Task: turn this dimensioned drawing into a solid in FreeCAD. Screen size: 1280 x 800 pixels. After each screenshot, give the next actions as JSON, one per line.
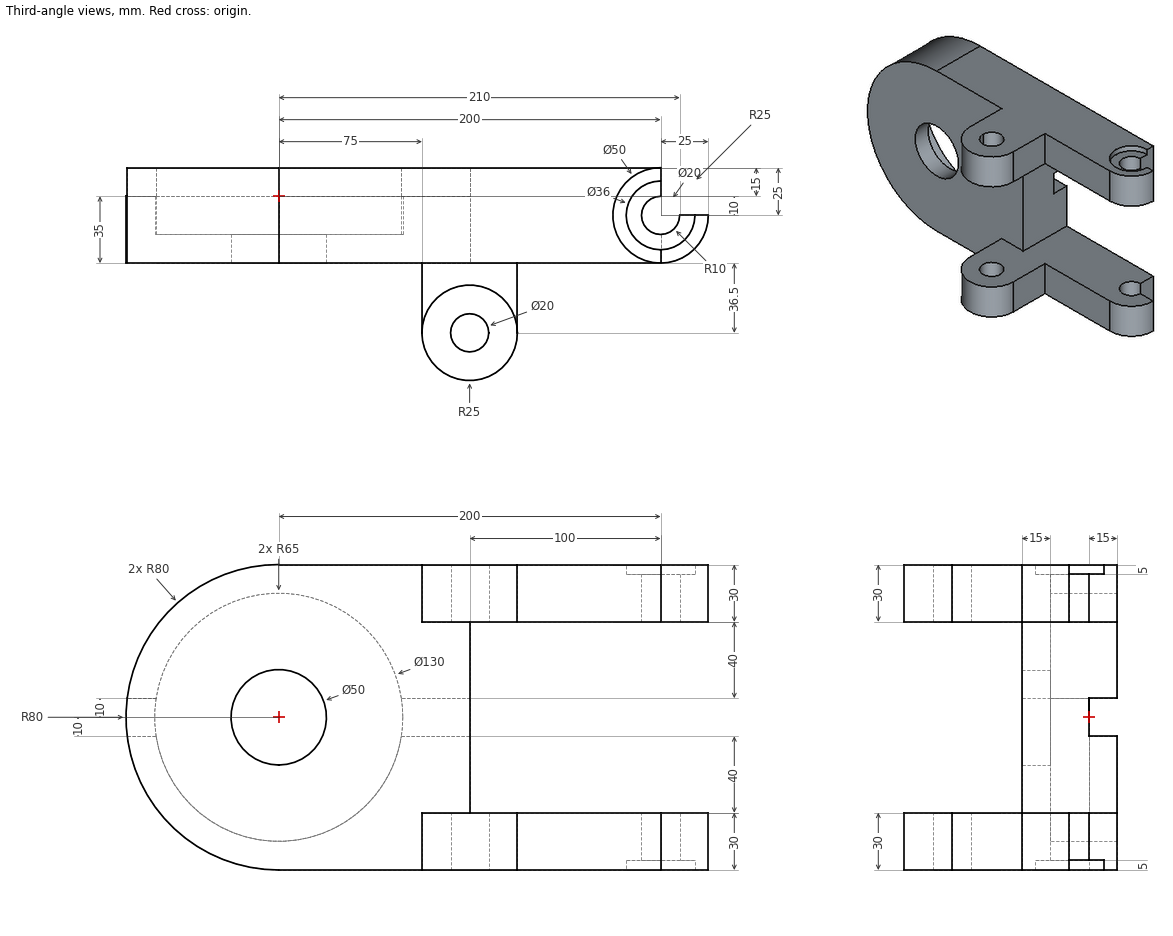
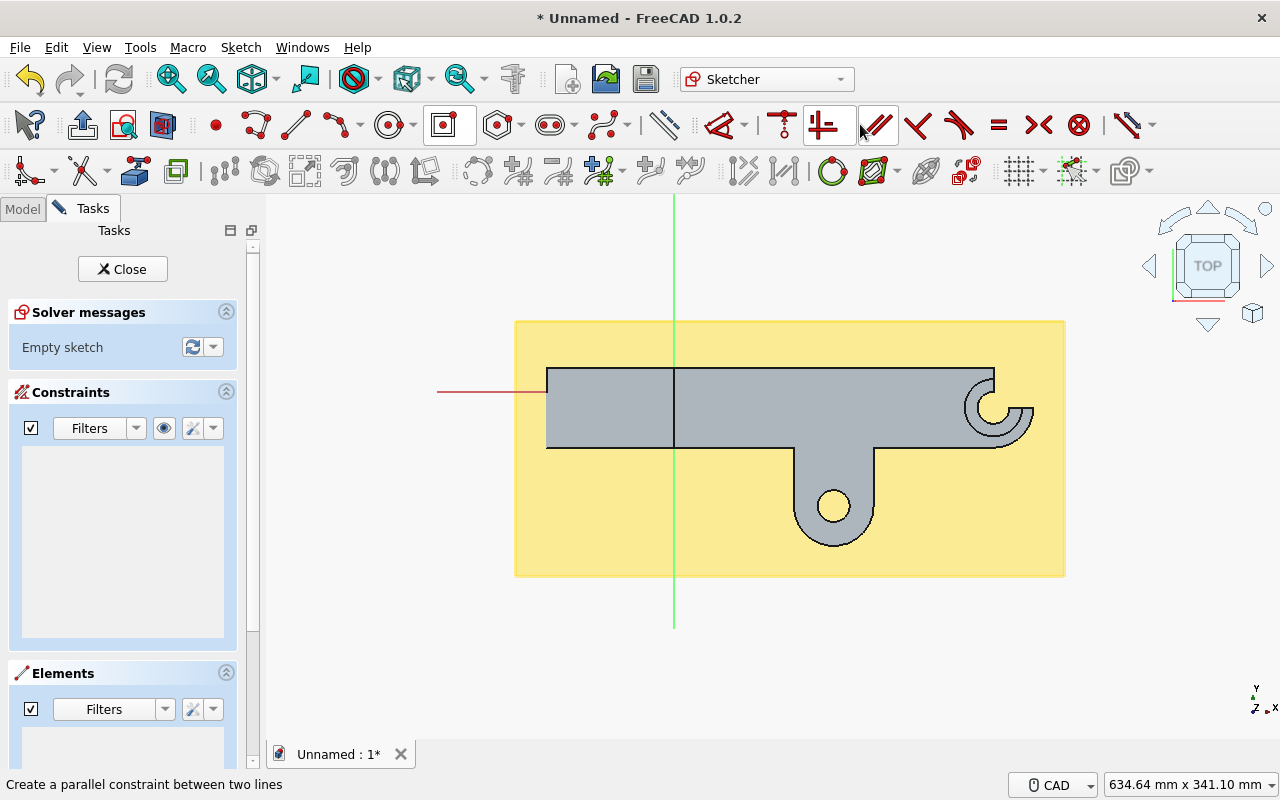
{"action": "key", "text": "q s"}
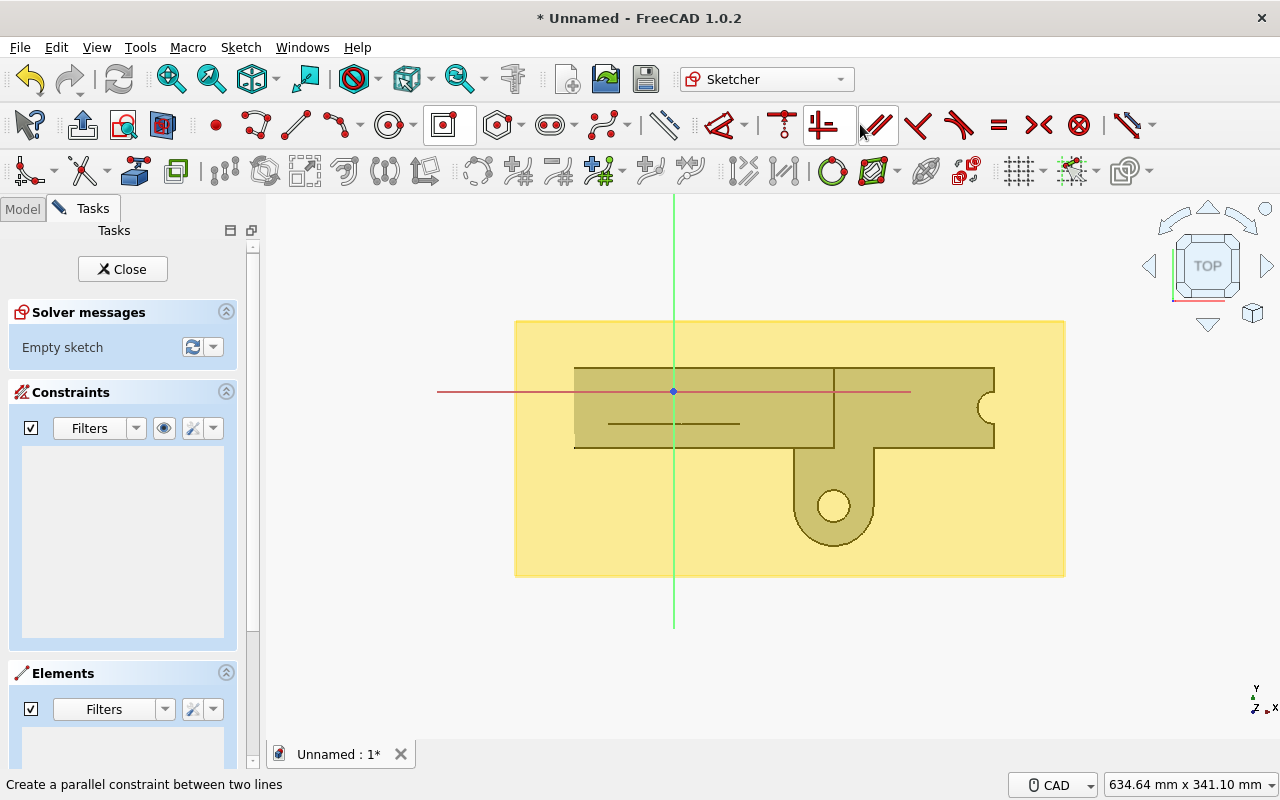
{"action": "scroll", "coordinate": [1052, 423], "scroll_direction": "up", "scroll_amount": 11}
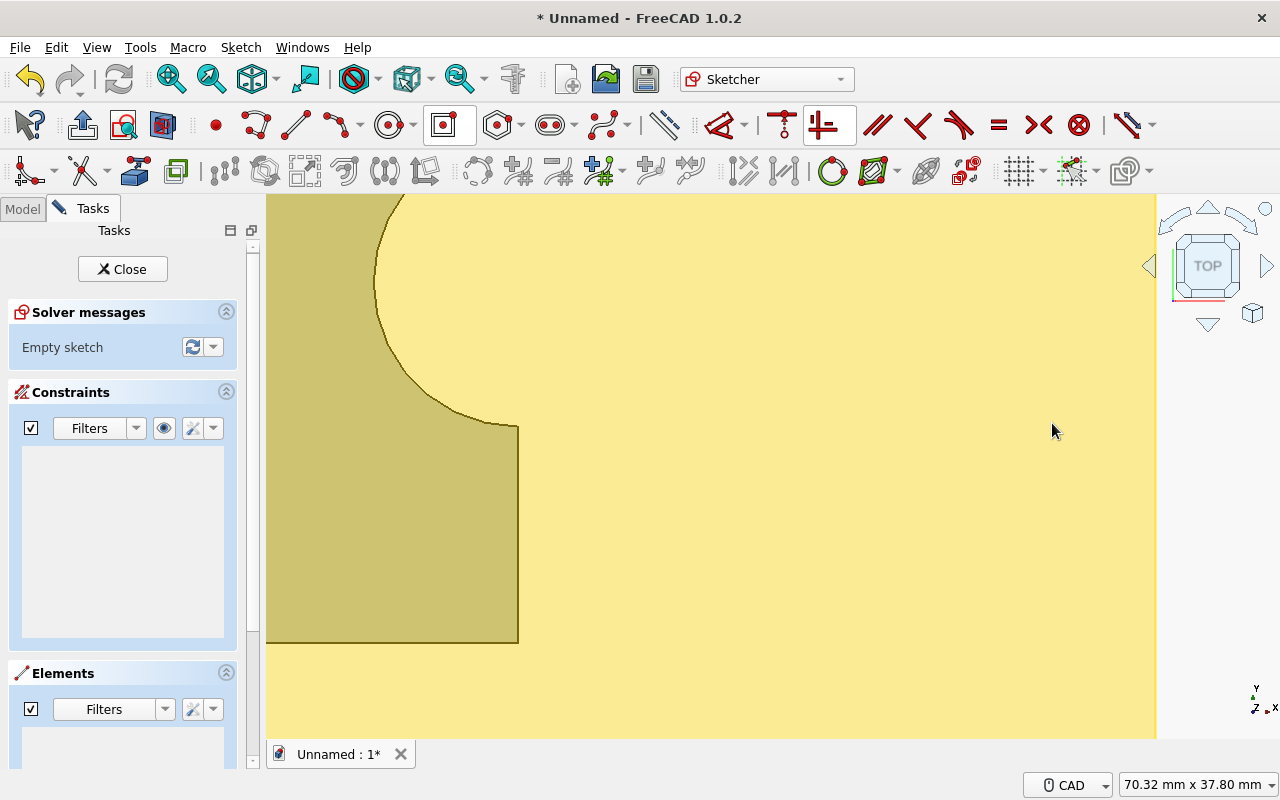
{"action": "key", "text": "g l"}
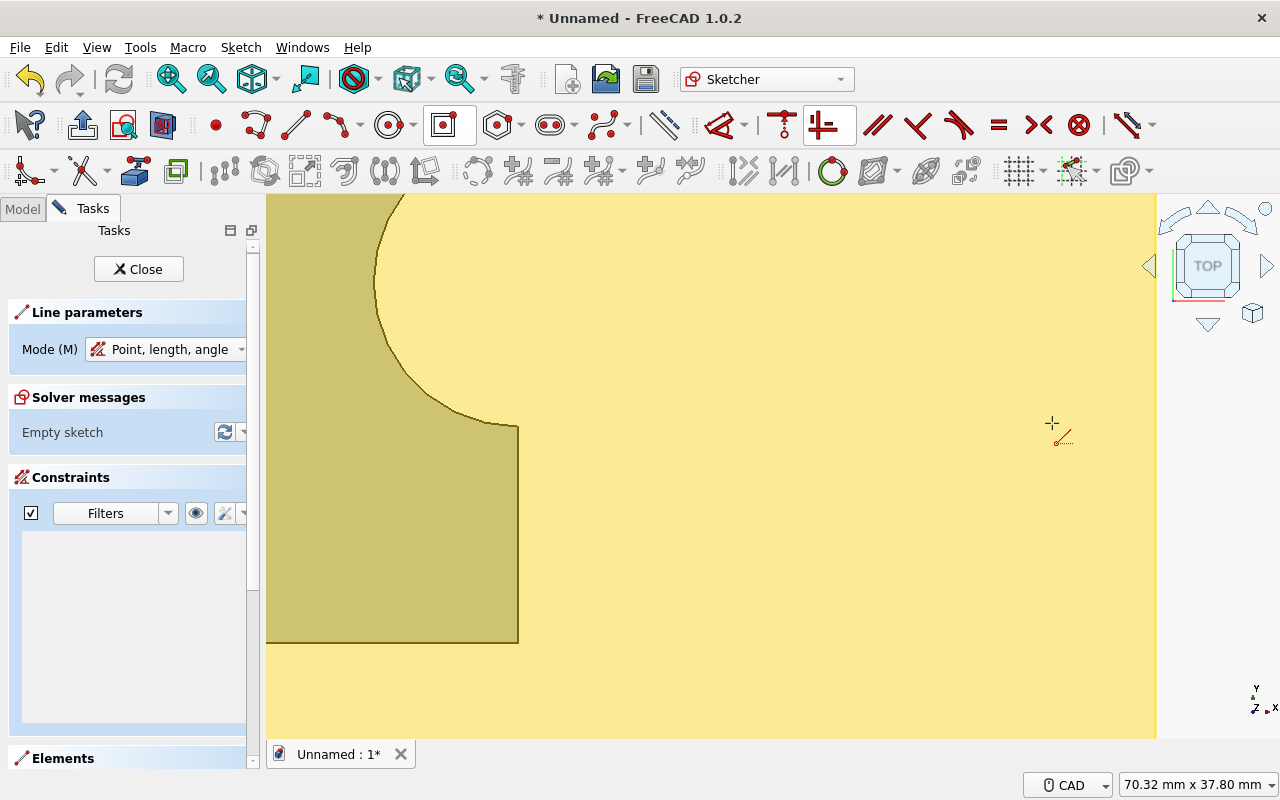
{"action": "left_click", "coordinate": [662, 282]}
{"action": "left_click", "coordinate": [878, 282]}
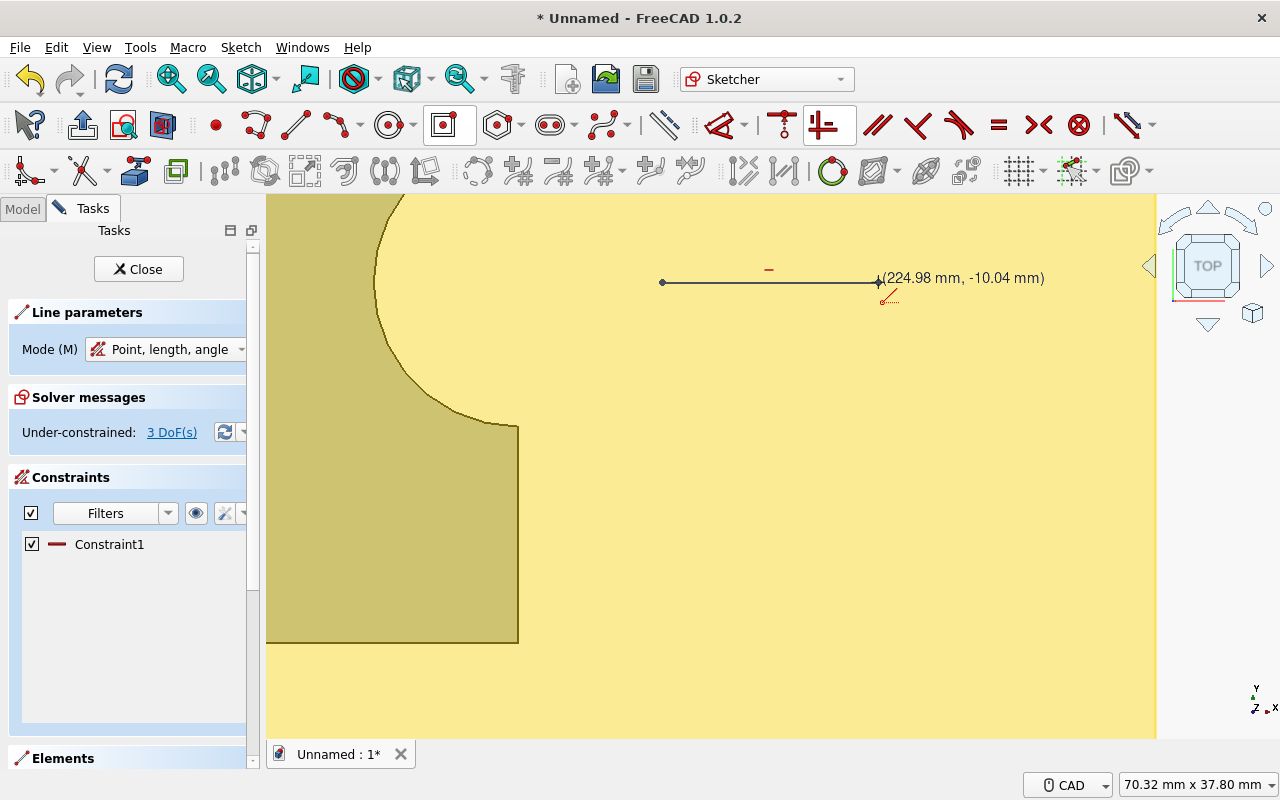
{"action": "left_click", "coordinate": [518, 643]}
{"action": "left_click", "coordinate": [518, 427]}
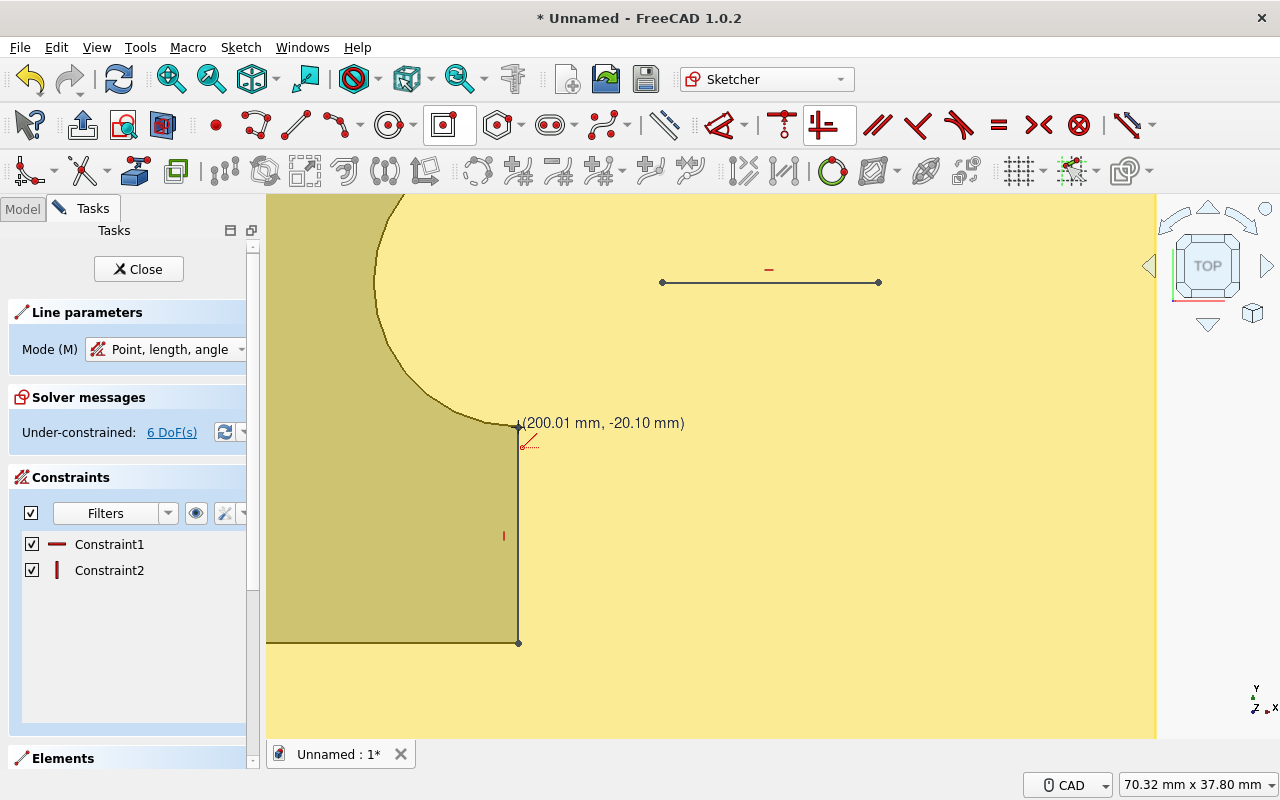
{"action": "key", "text": "g 3 a"}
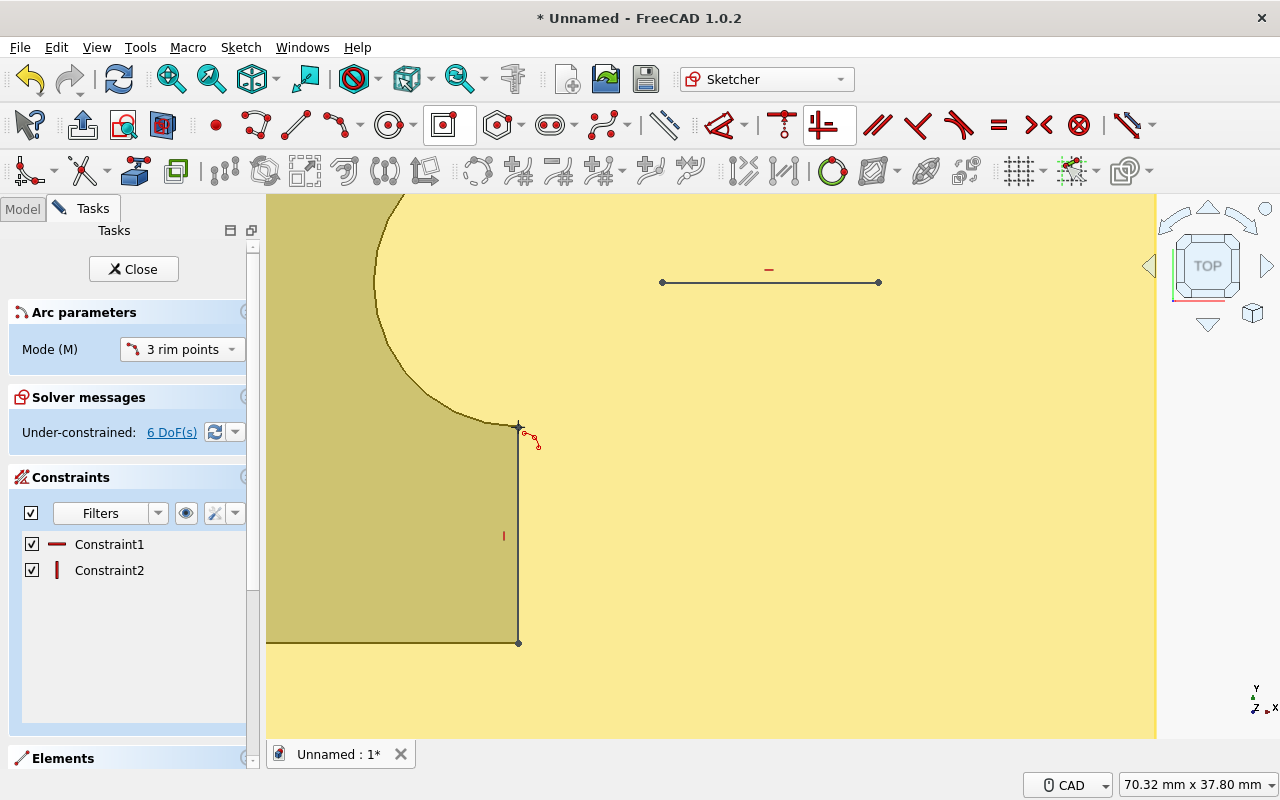
{"action": "left_click", "coordinate": [878, 283]}
{"action": "left_click", "coordinate": [518, 644]}
{"action": "left_click", "coordinate": [773, 537]}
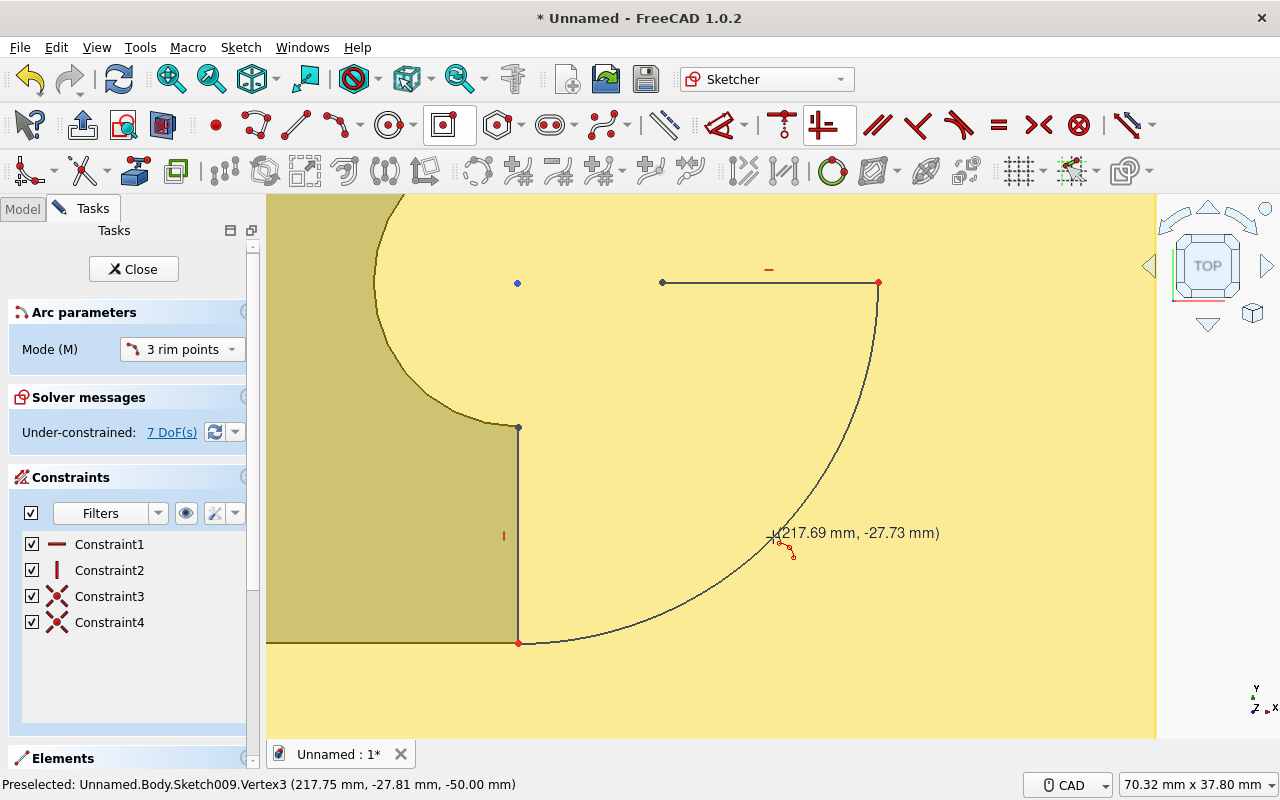
{"action": "left_click", "coordinate": [518, 428]}
{"action": "left_click", "coordinate": [662, 283]}
{"action": "left_click", "coordinate": [620, 384]}
{"action": "key", "text": "Escape"}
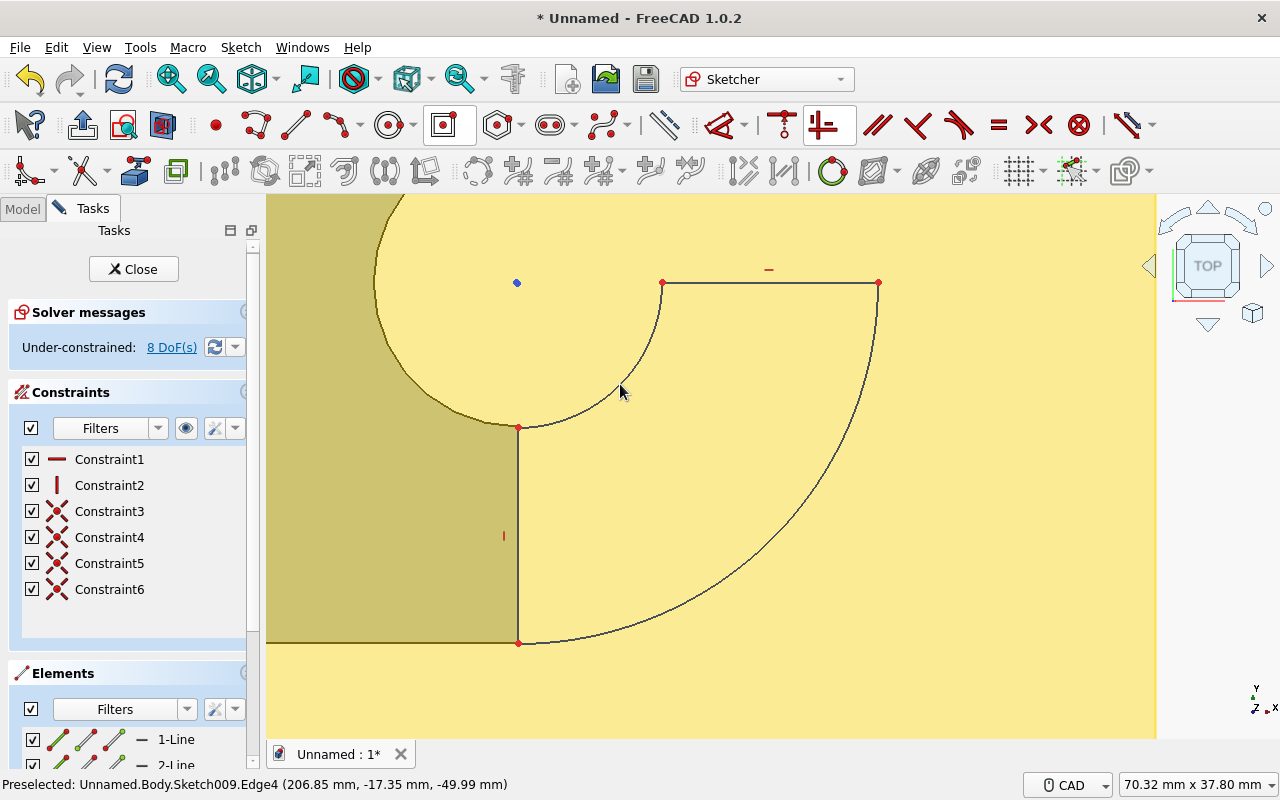
{"action": "left_click", "coordinate": [682, 605]}